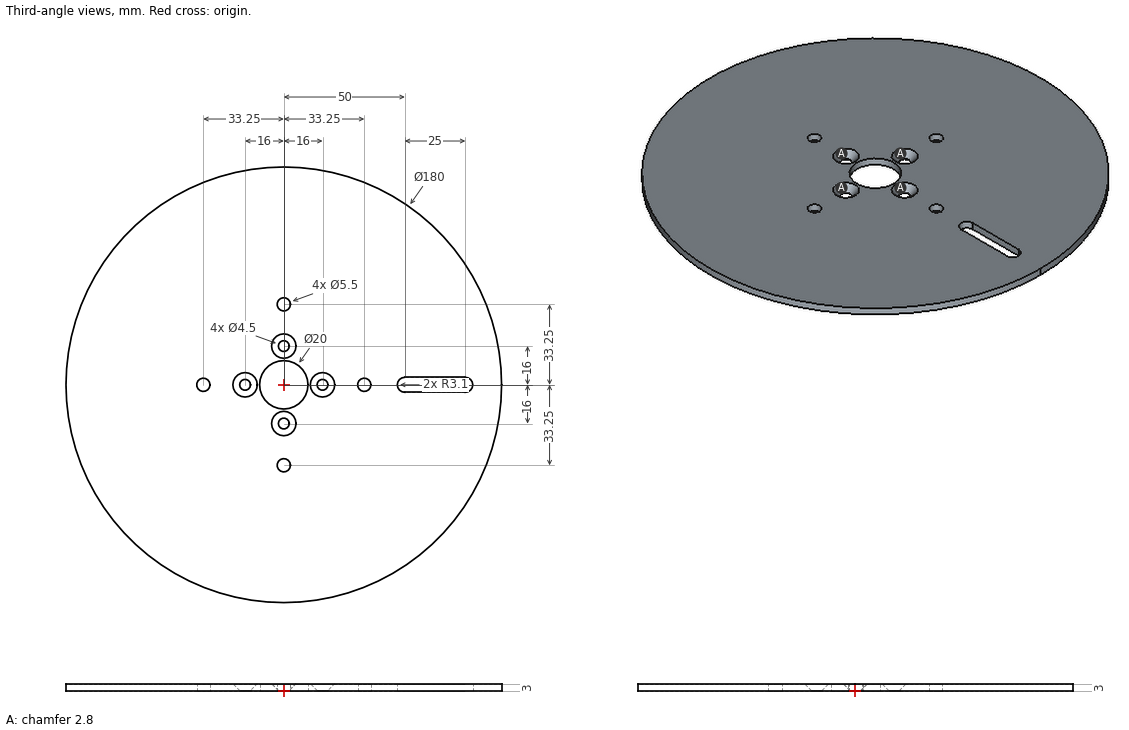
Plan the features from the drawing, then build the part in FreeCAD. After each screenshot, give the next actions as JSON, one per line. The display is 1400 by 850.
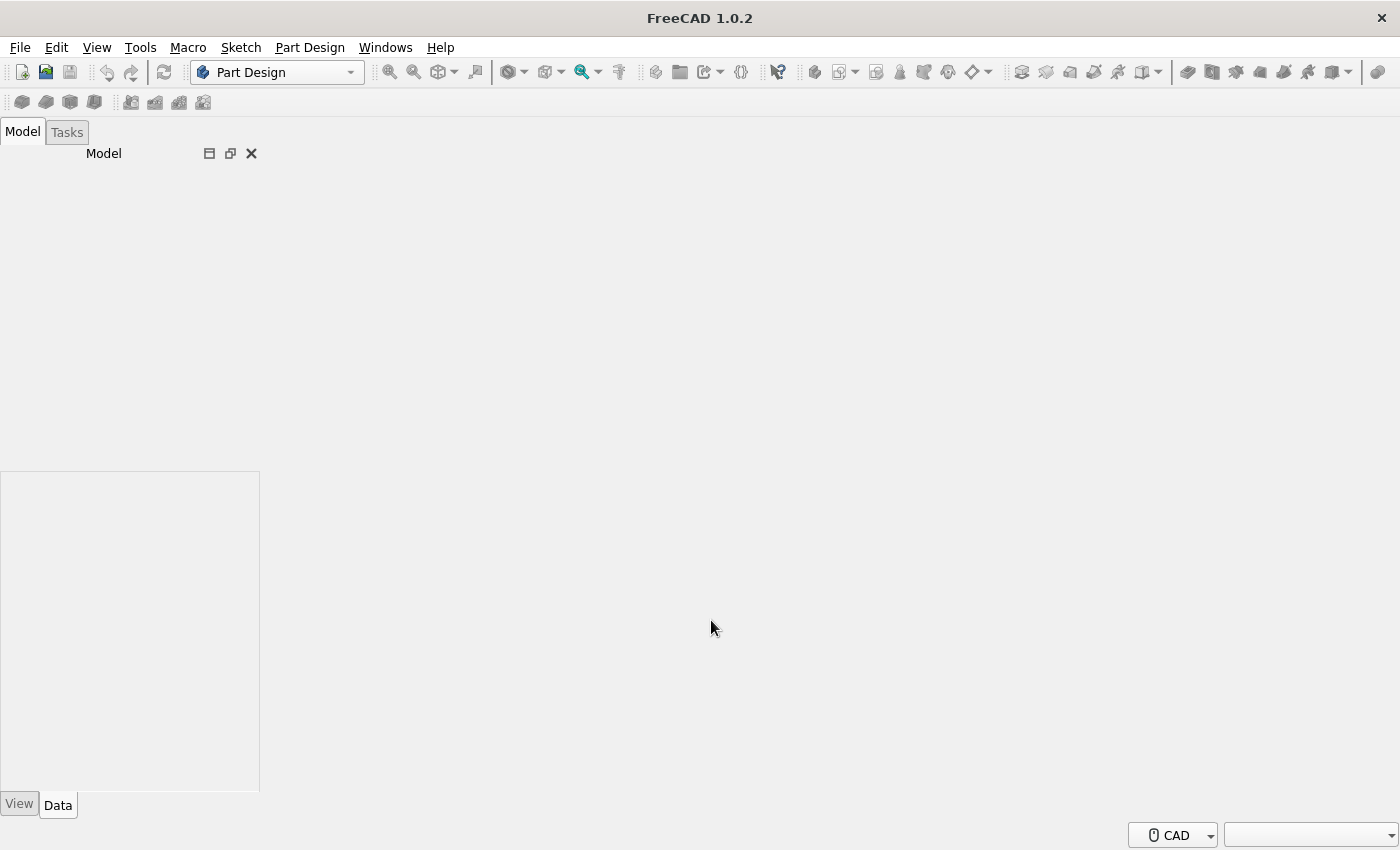
{"action": "left_click", "coordinate": [22, 72]}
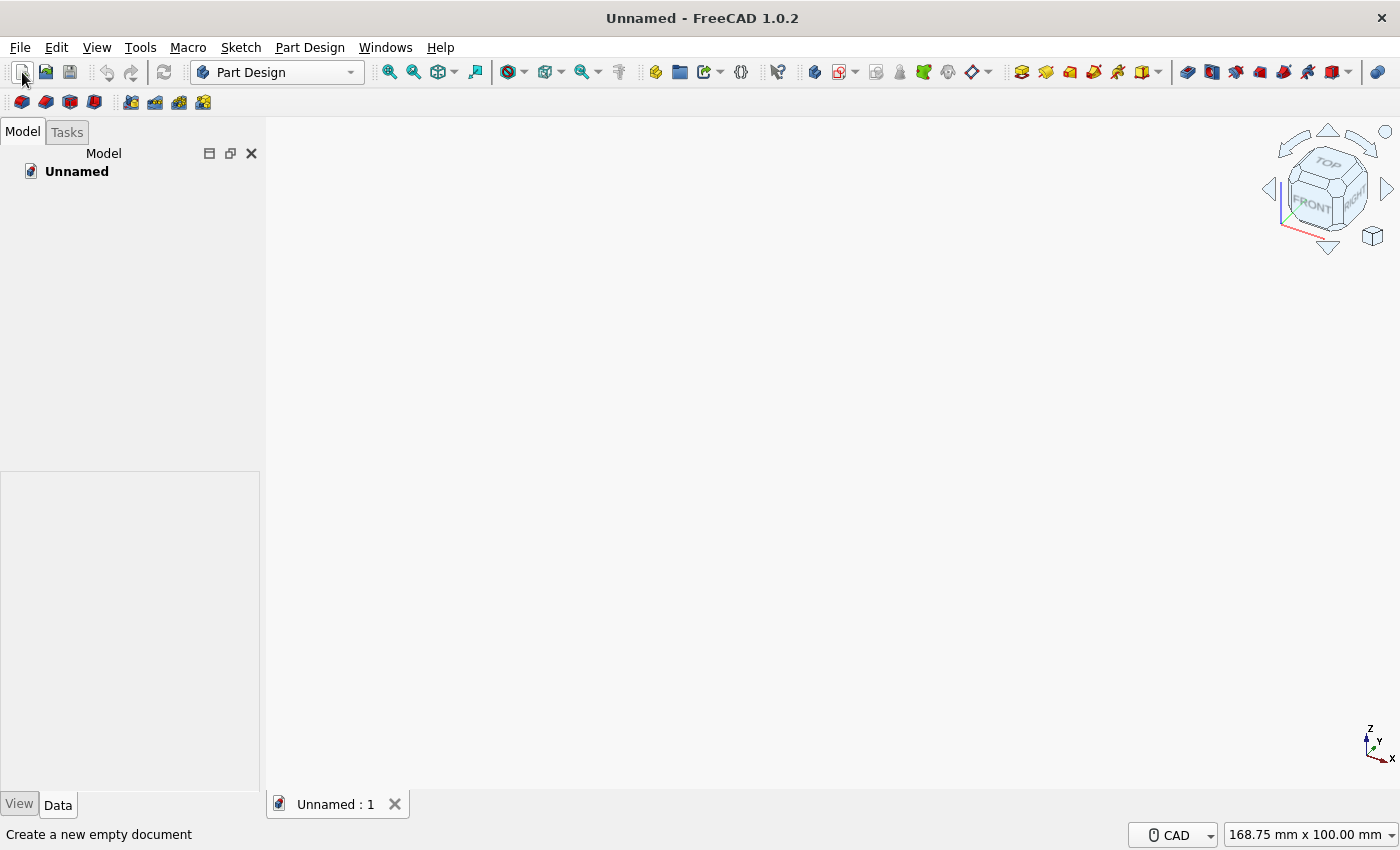
{"action": "left_click", "coordinate": [840, 72]}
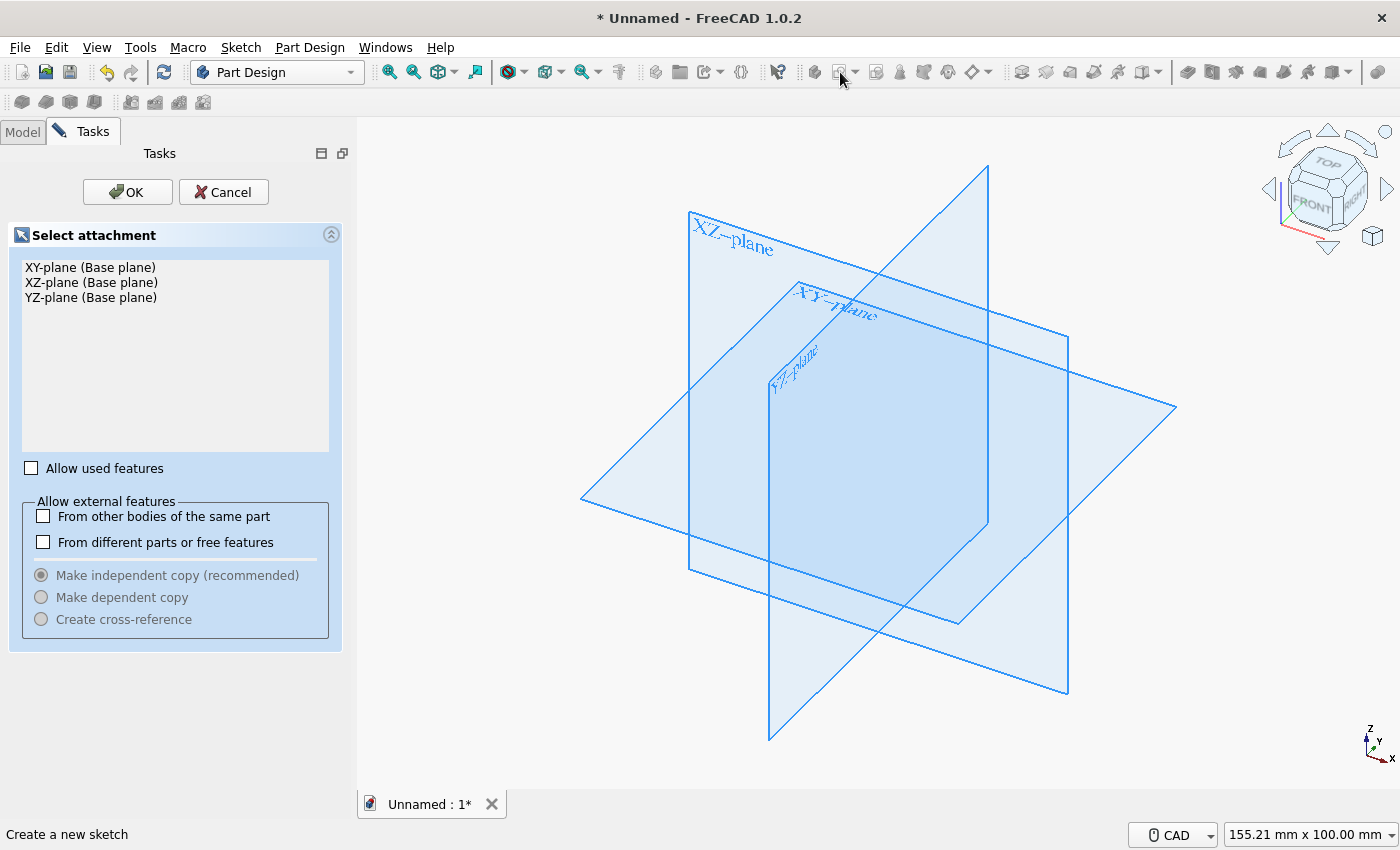
{"action": "left_click", "coordinate": [82, 268]}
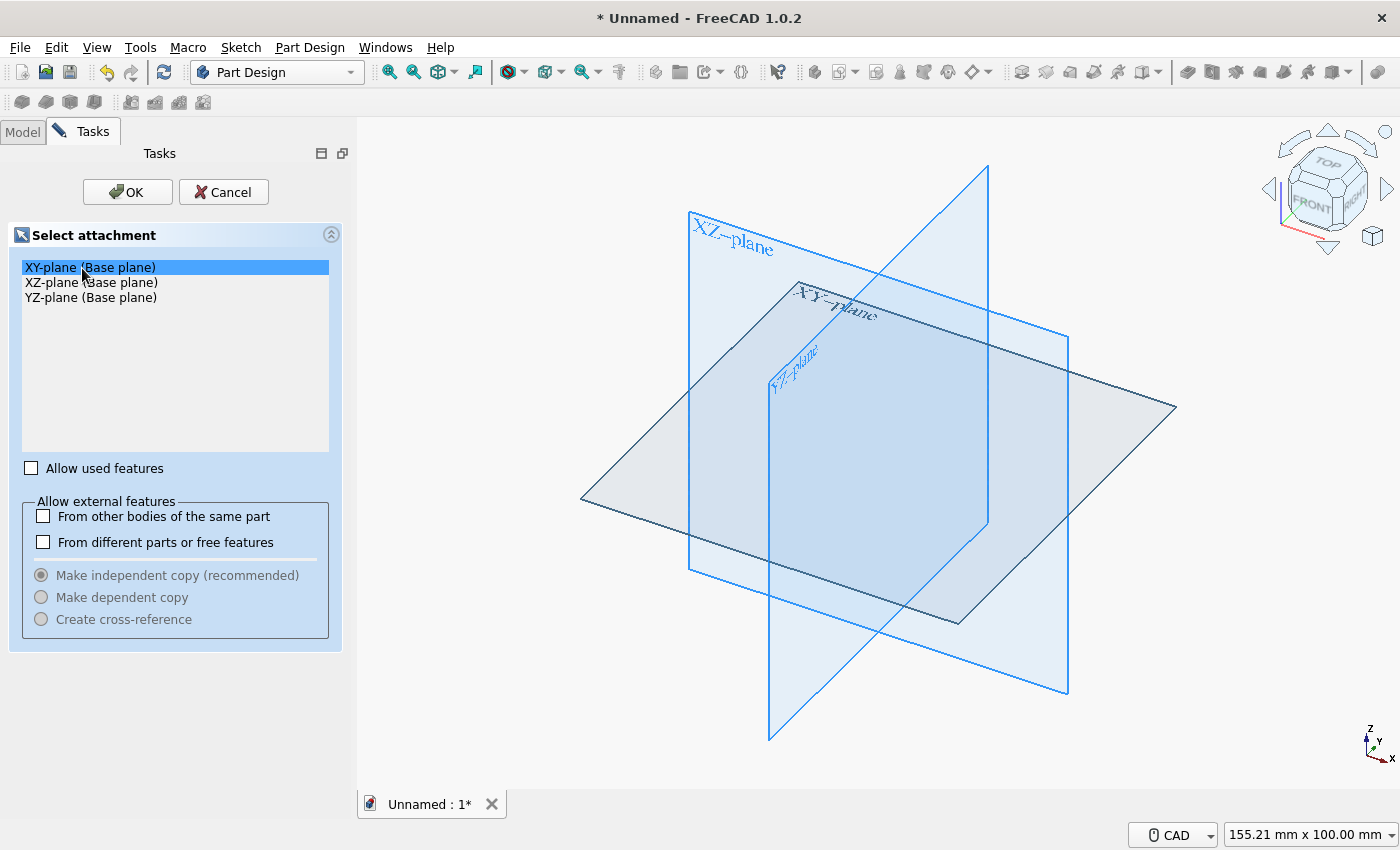
{"action": "left_click", "coordinate": [128, 192]}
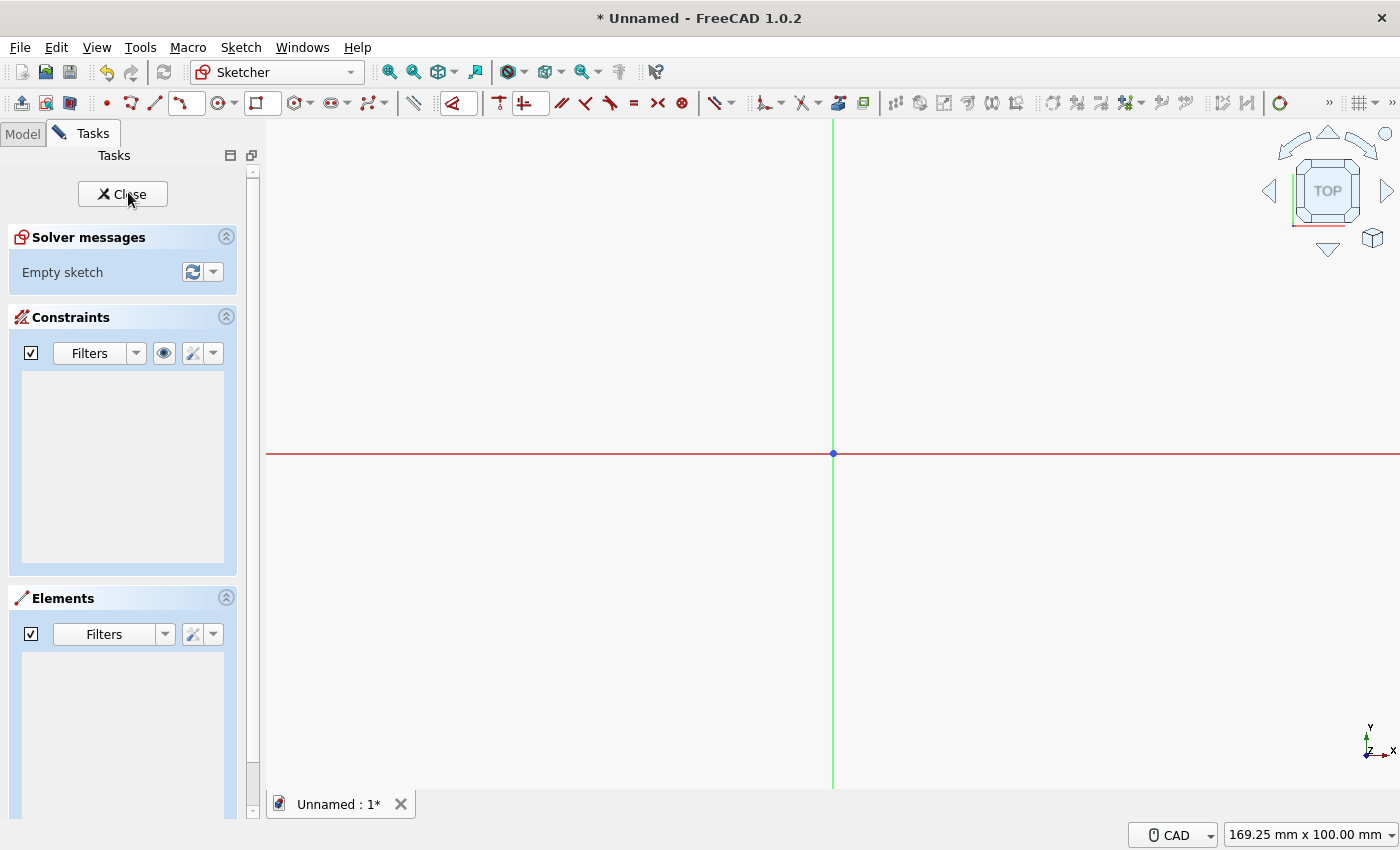
{"action": "scroll", "coordinate": [725, 454], "scroll_direction": "down", "scroll_amount": 5}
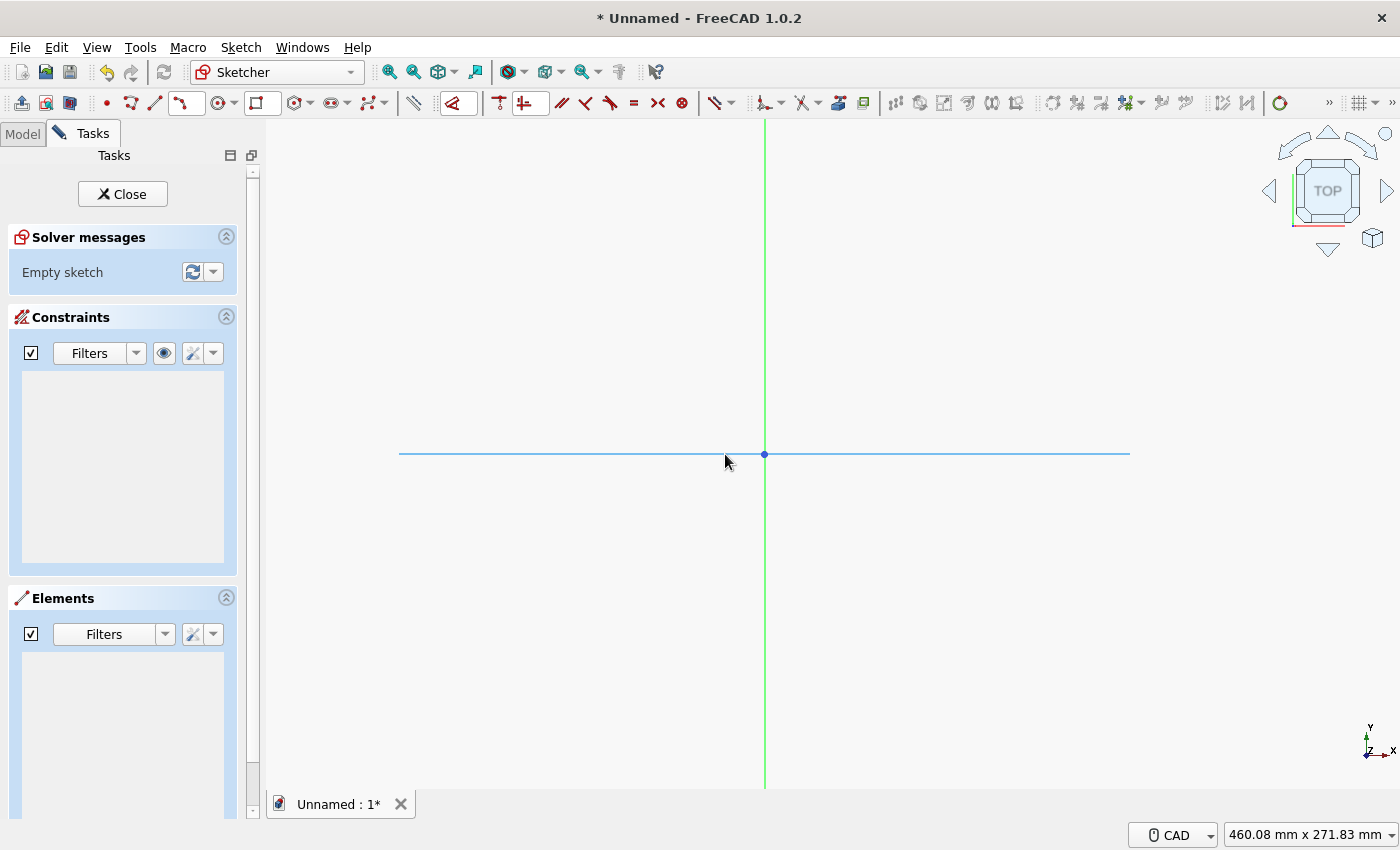
{"action": "left_click", "coordinate": [218, 104]}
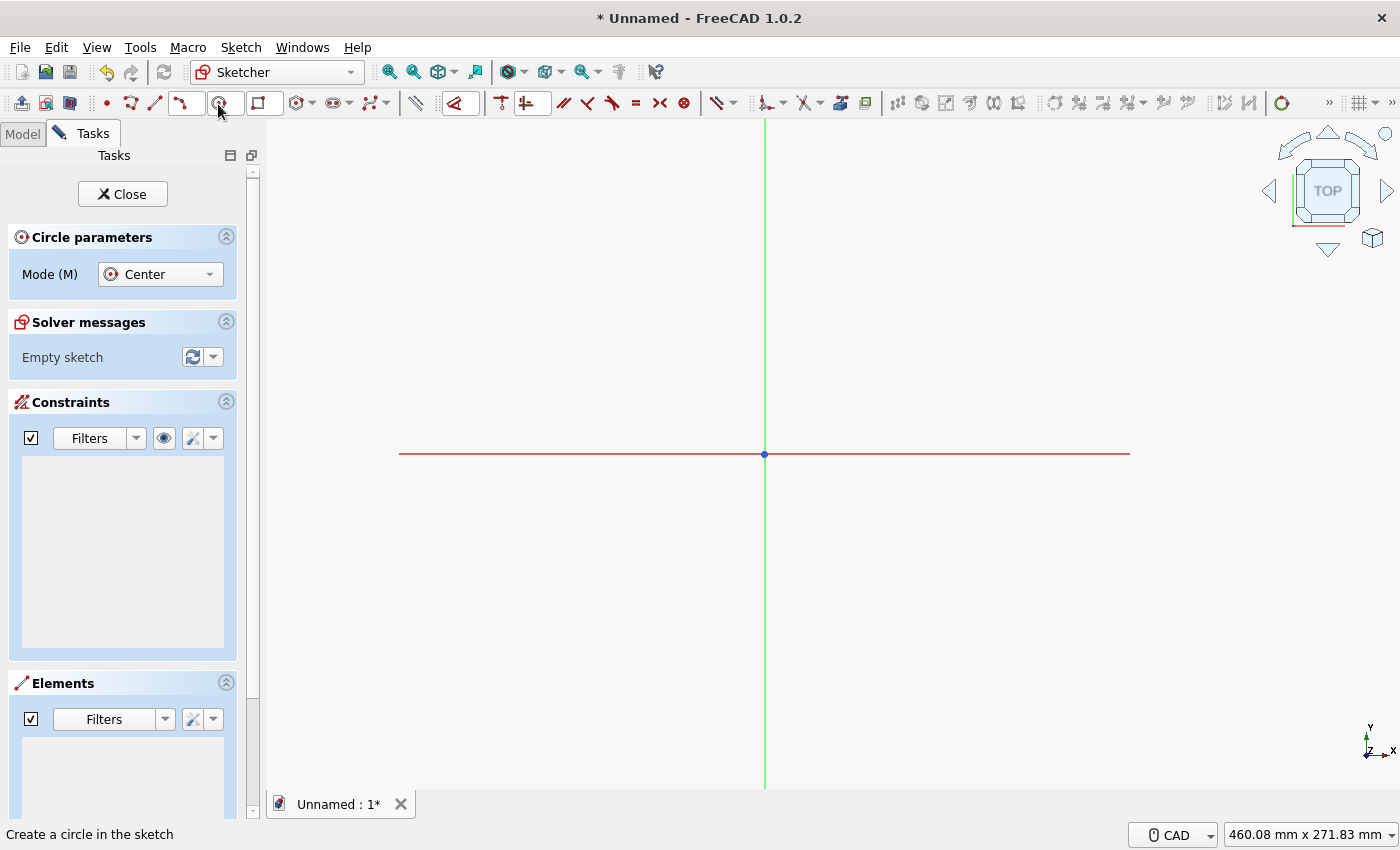
{"action": "left_click", "coordinate": [765, 454]}
{"action": "left_click", "coordinate": [922, 297]}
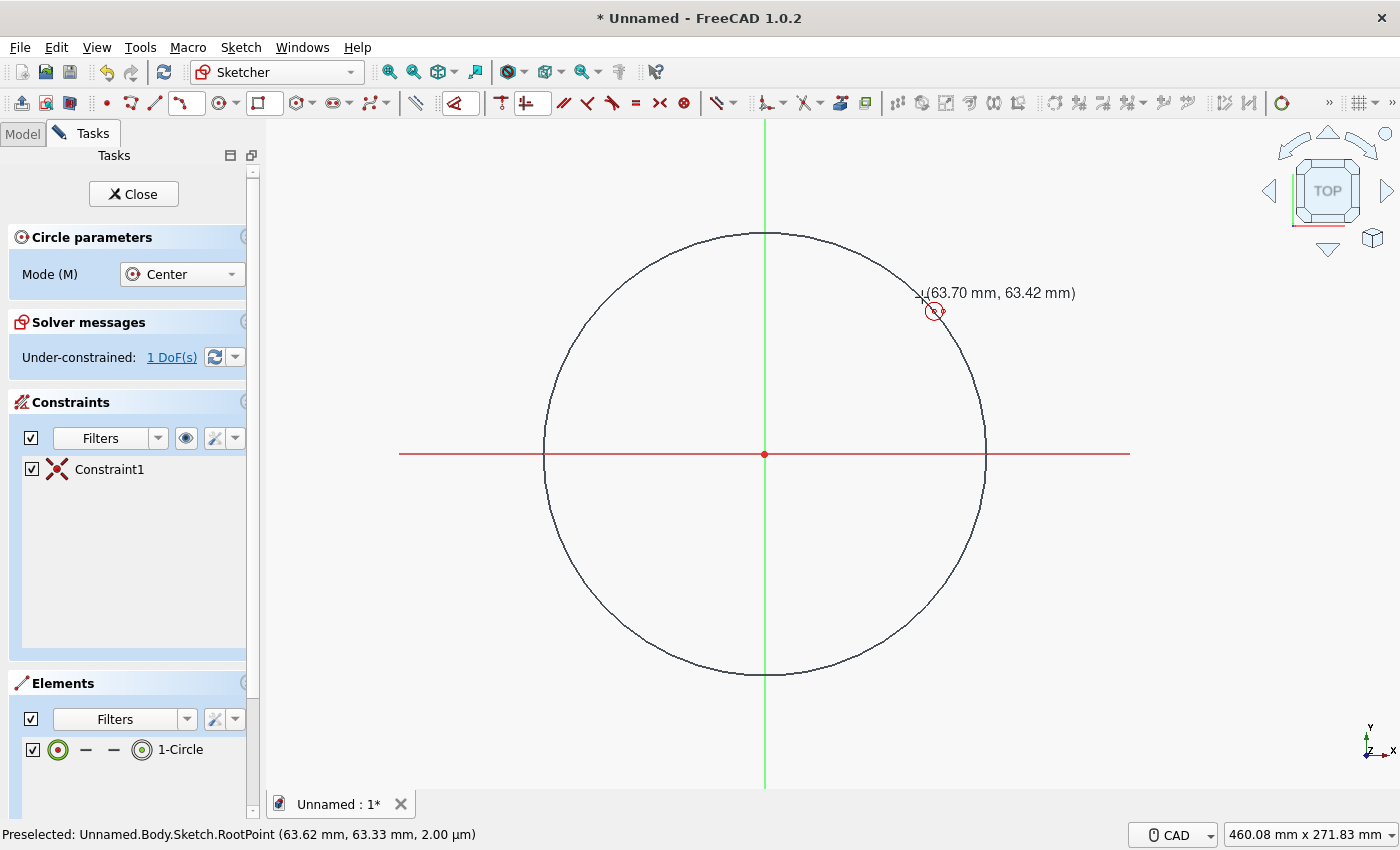
{"action": "left_click", "coordinate": [765, 454]}
{"action": "left_click", "coordinate": [782, 437]}
{"action": "key", "text": "Escape"}